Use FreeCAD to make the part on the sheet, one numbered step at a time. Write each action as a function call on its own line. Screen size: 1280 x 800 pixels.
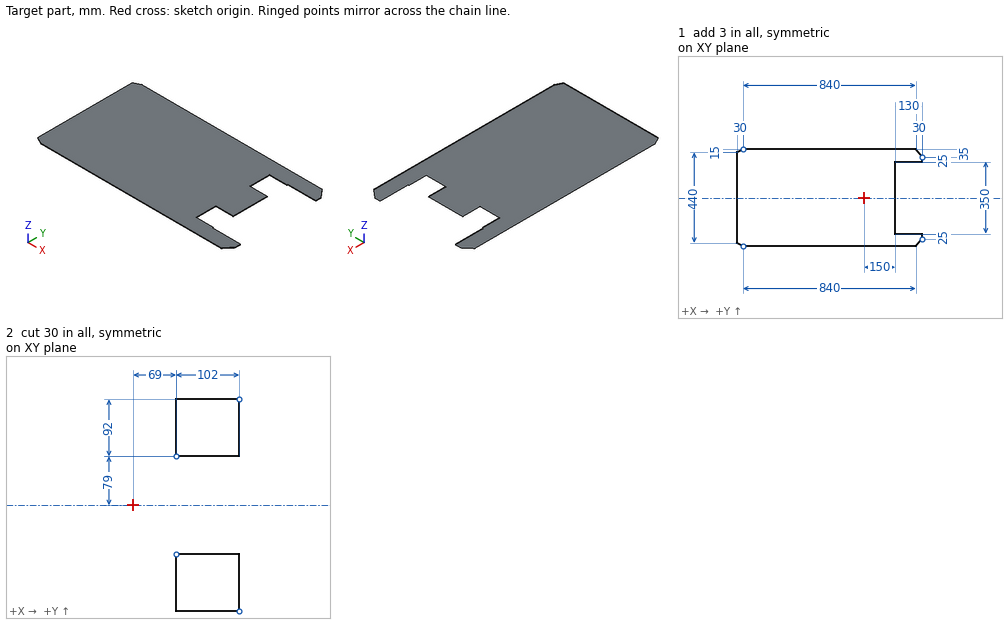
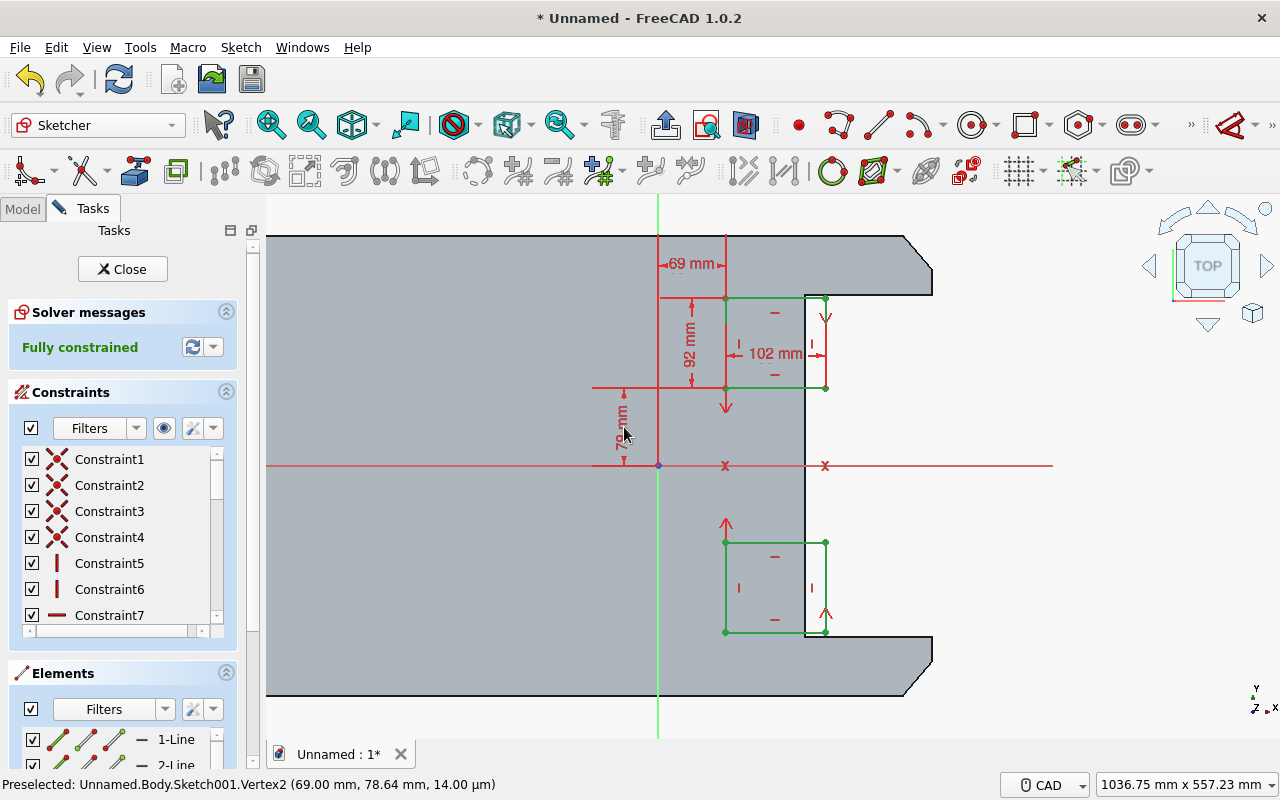
click(123, 269)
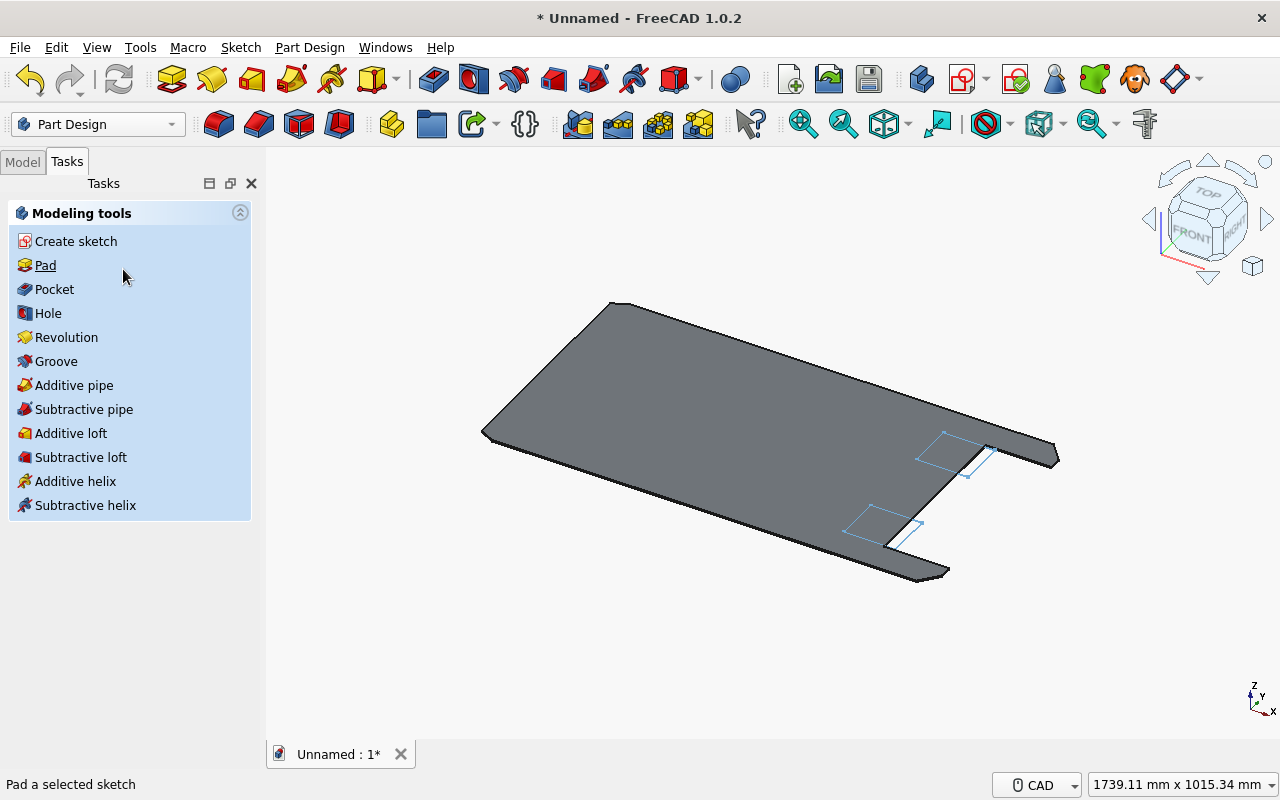
click(434, 80)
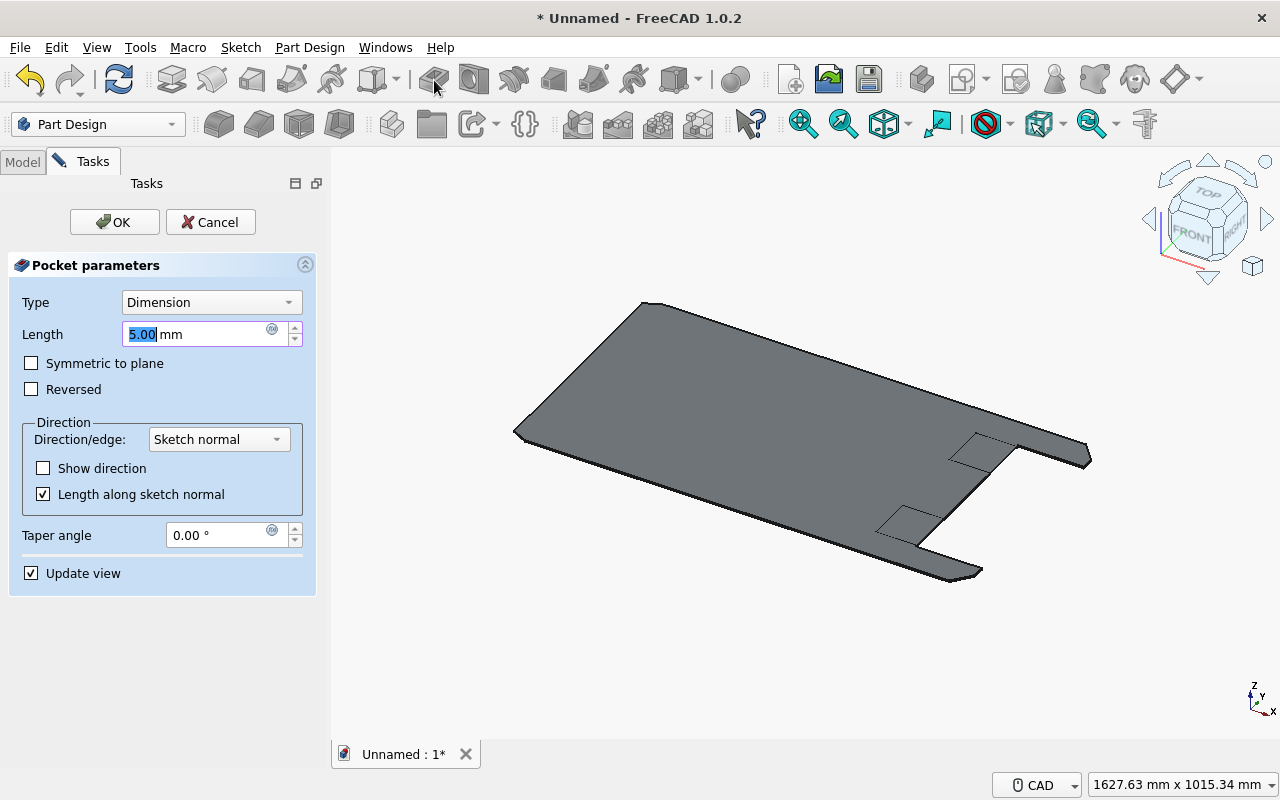
text(30)
key(Tab)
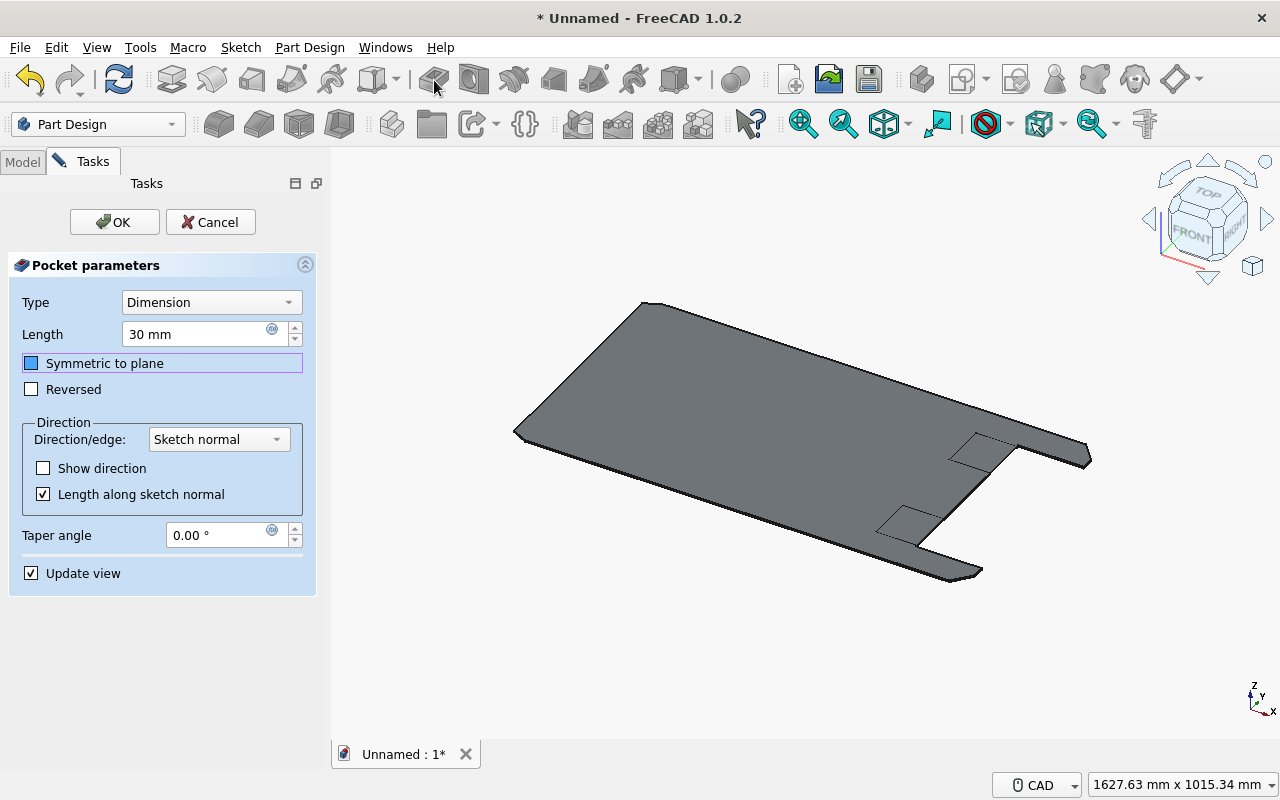
click(30, 363)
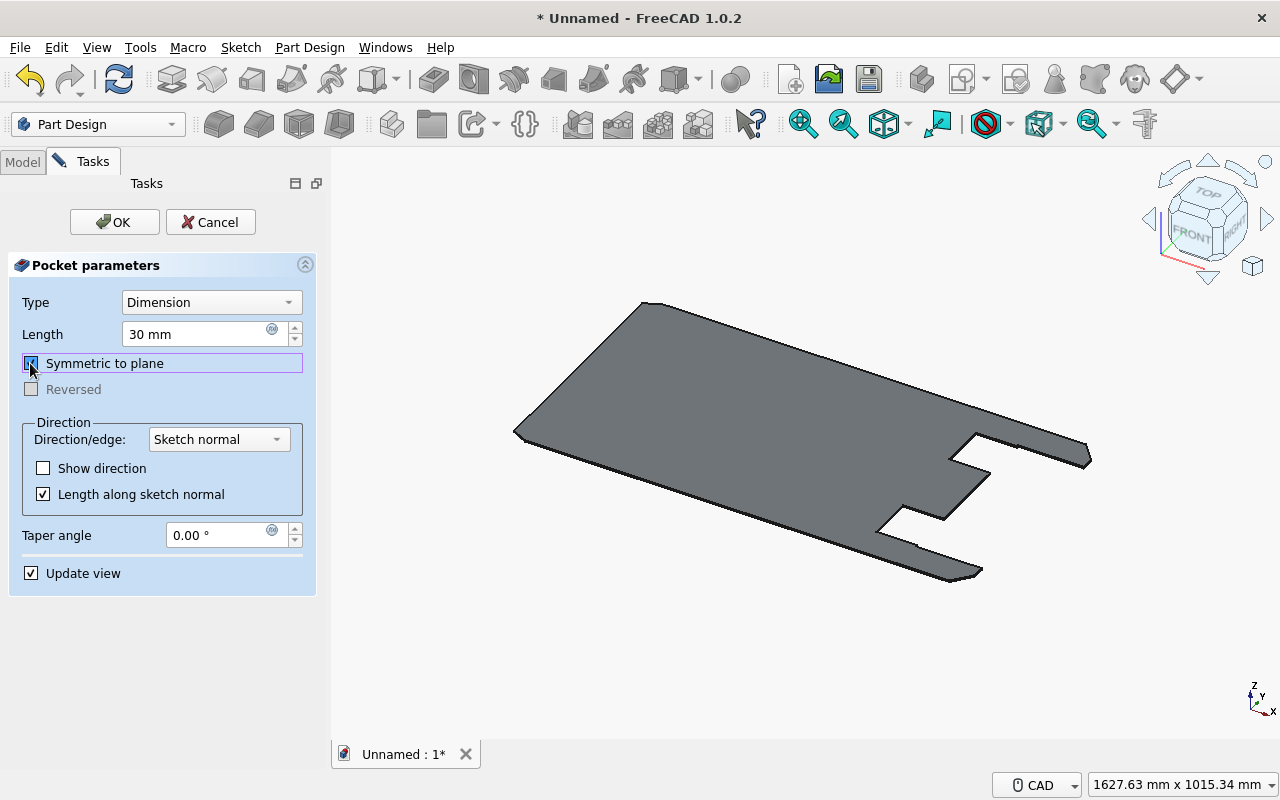
click(115, 222)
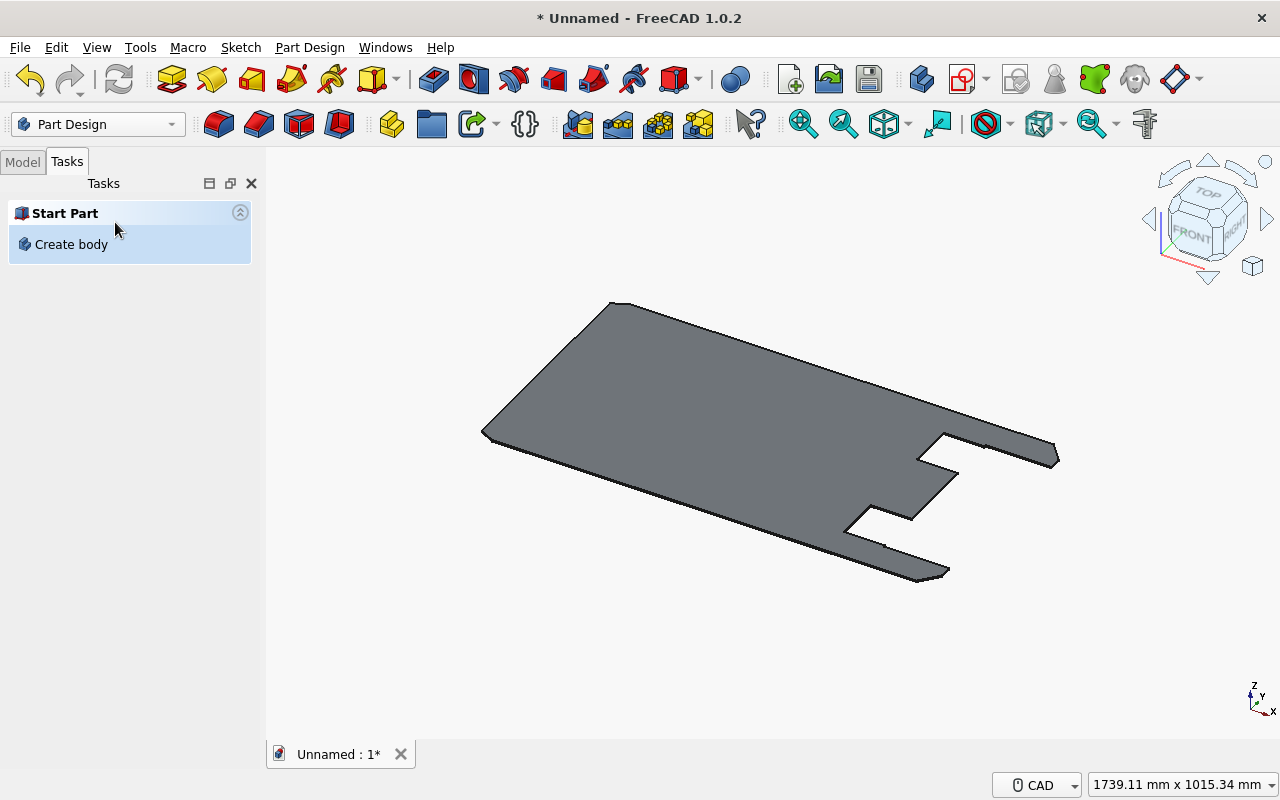
key(0)